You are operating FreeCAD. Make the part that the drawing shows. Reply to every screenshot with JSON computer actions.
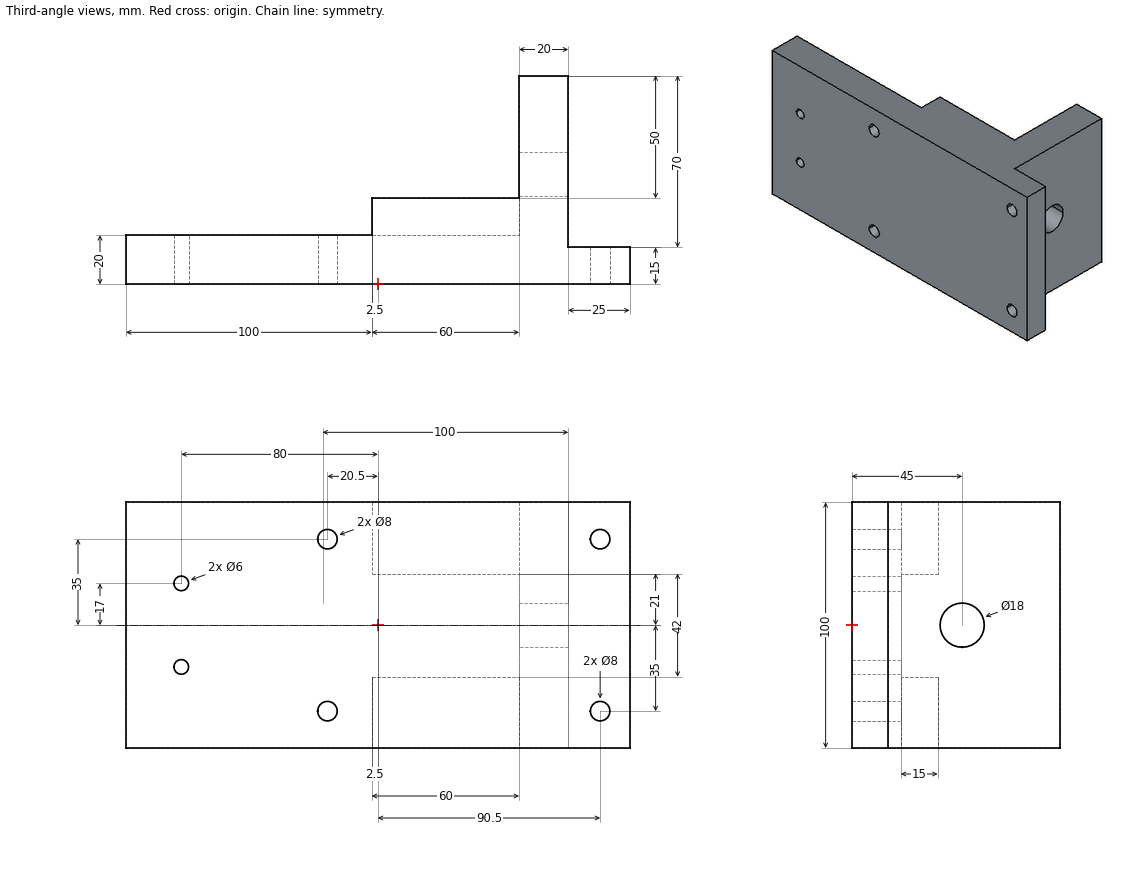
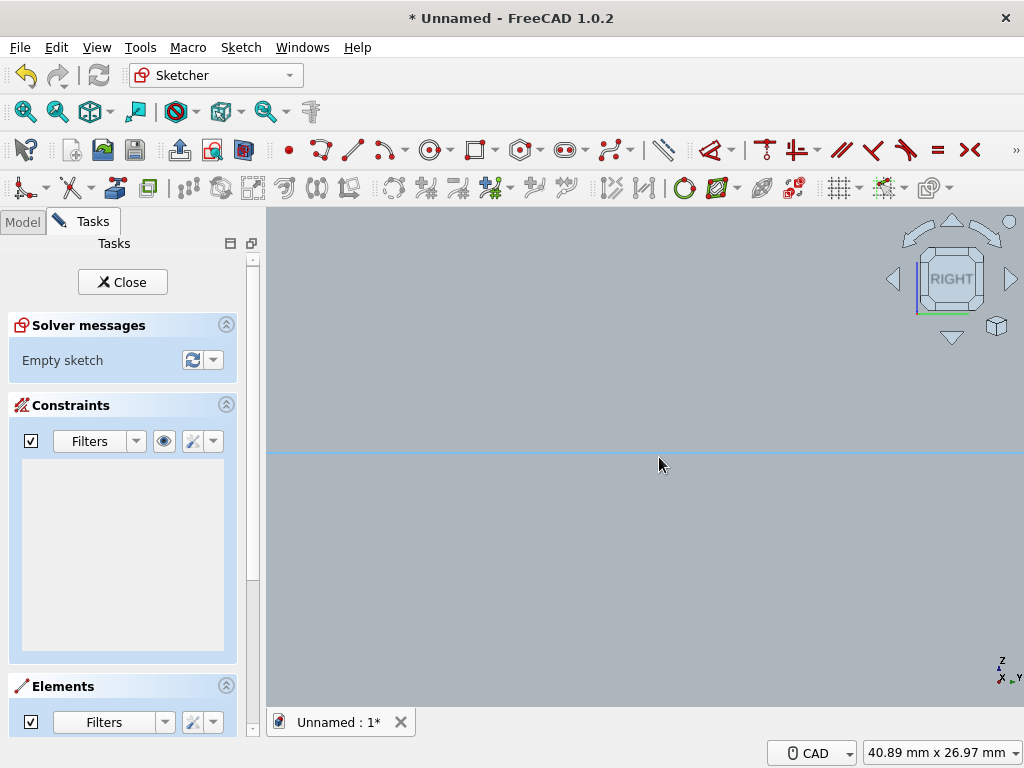
{"action": "left_click", "coordinate": [430, 150]}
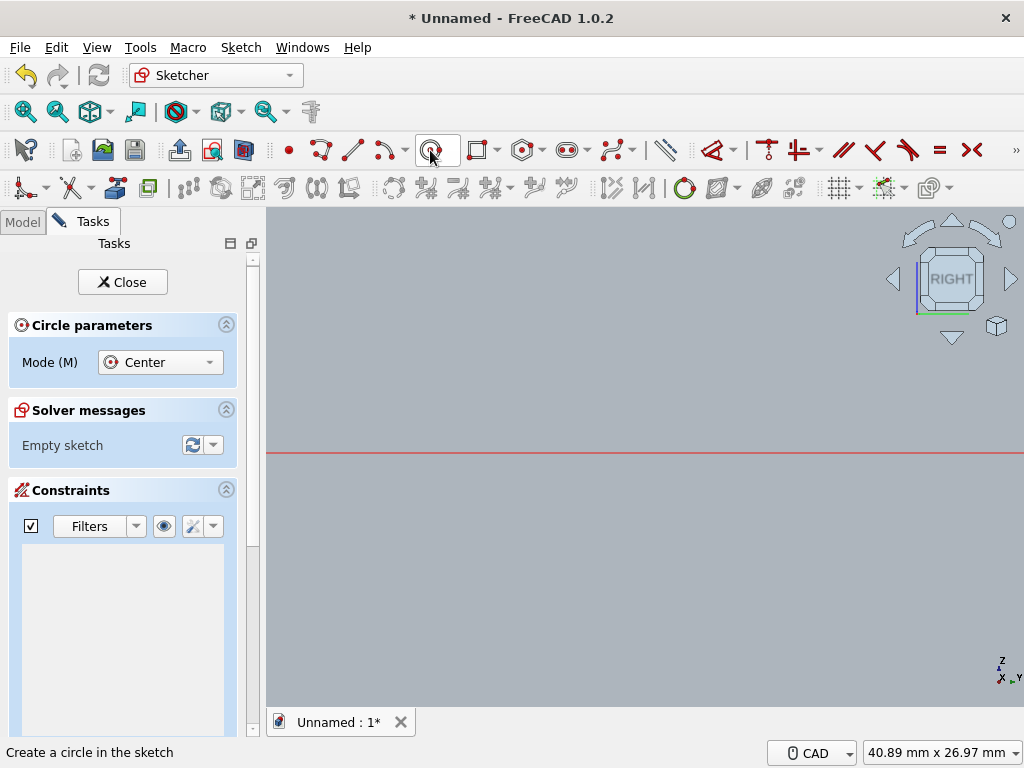
{"action": "left_click", "coordinate": [575, 453]}
{"action": "left_click", "coordinate": [693, 335]}
{"action": "key", "text": "Escape"}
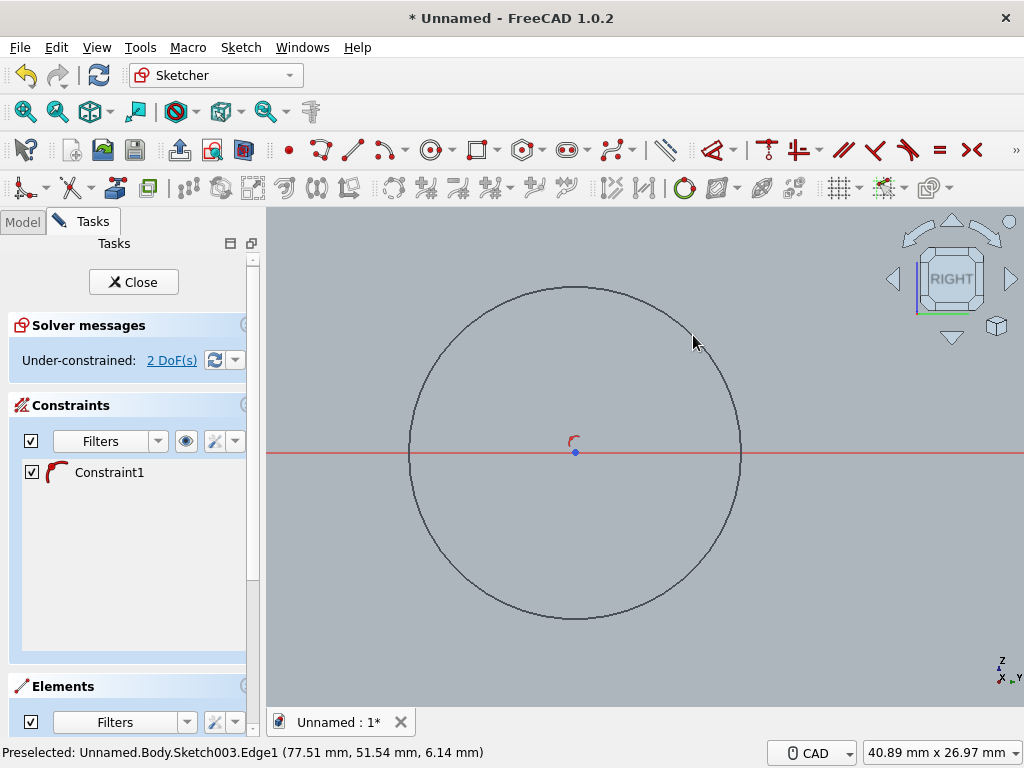
{"action": "left_click", "coordinate": [712, 150]}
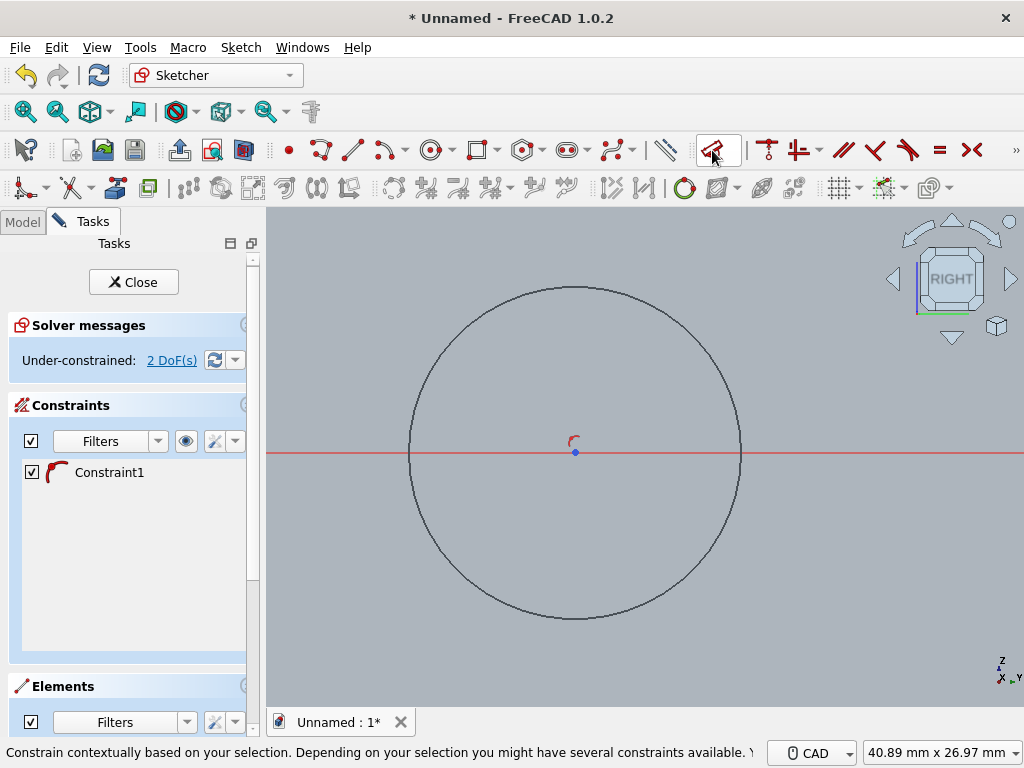
{"action": "left_click", "coordinate": [692, 335]}
{"action": "left_click", "coordinate": [715, 312]}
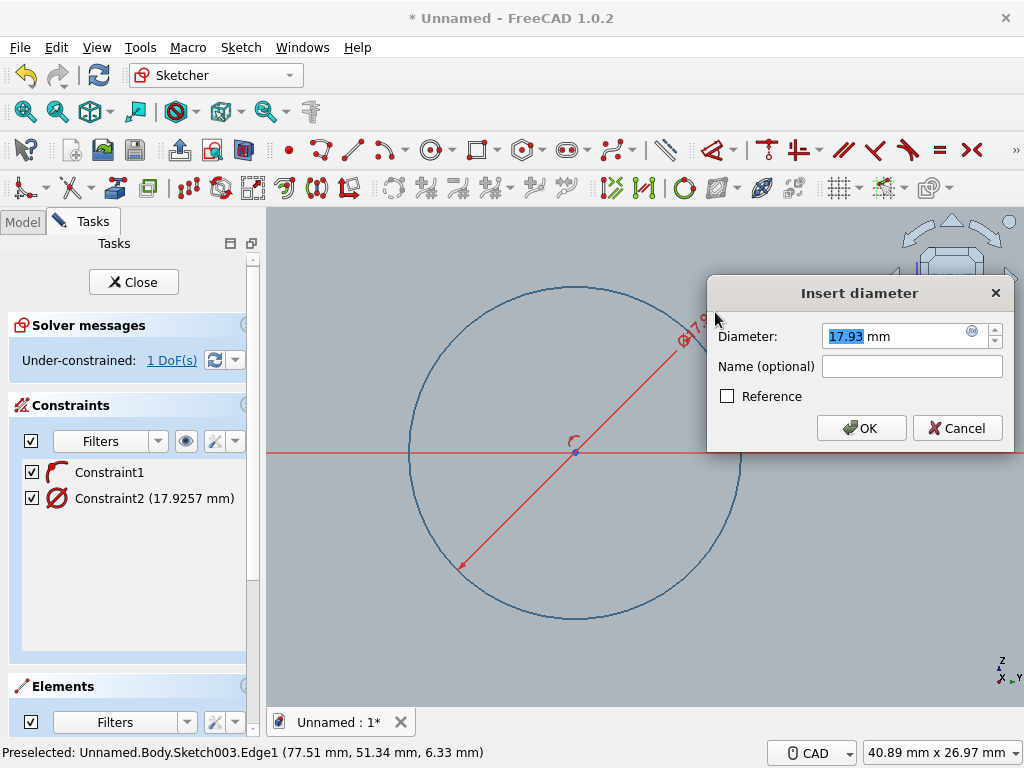
{"action": "type", "text": "18"}
{"action": "key", "text": "Return"}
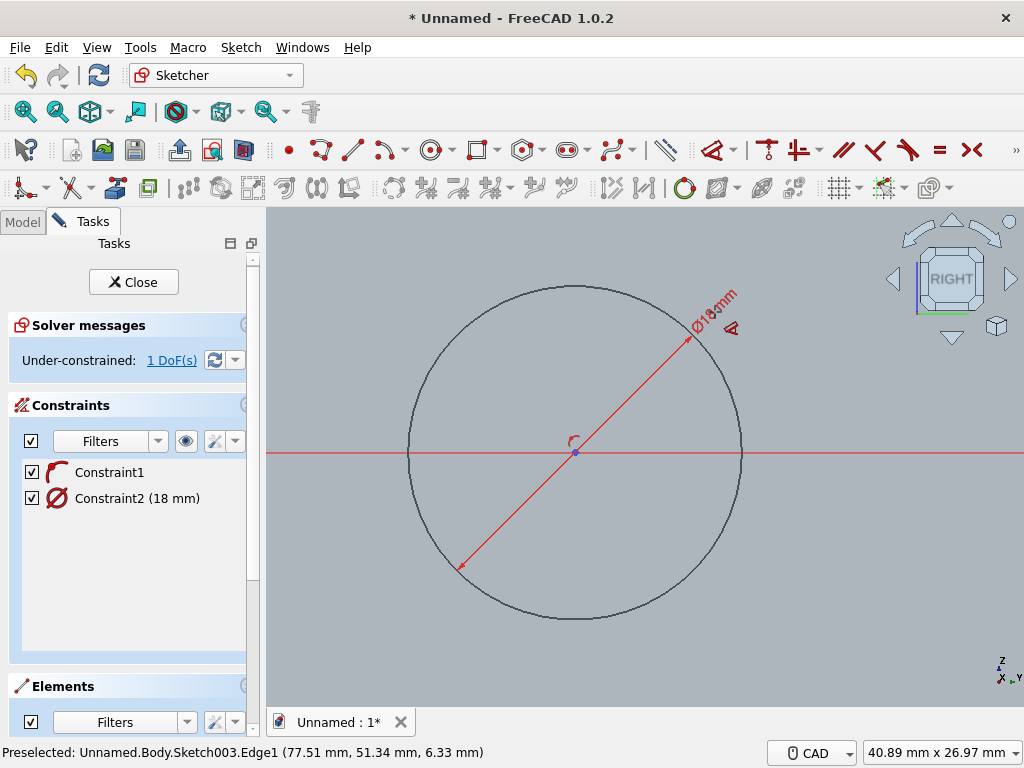
{"action": "left_click", "coordinate": [575, 453]}
{"action": "left_click", "coordinate": [434, 487]}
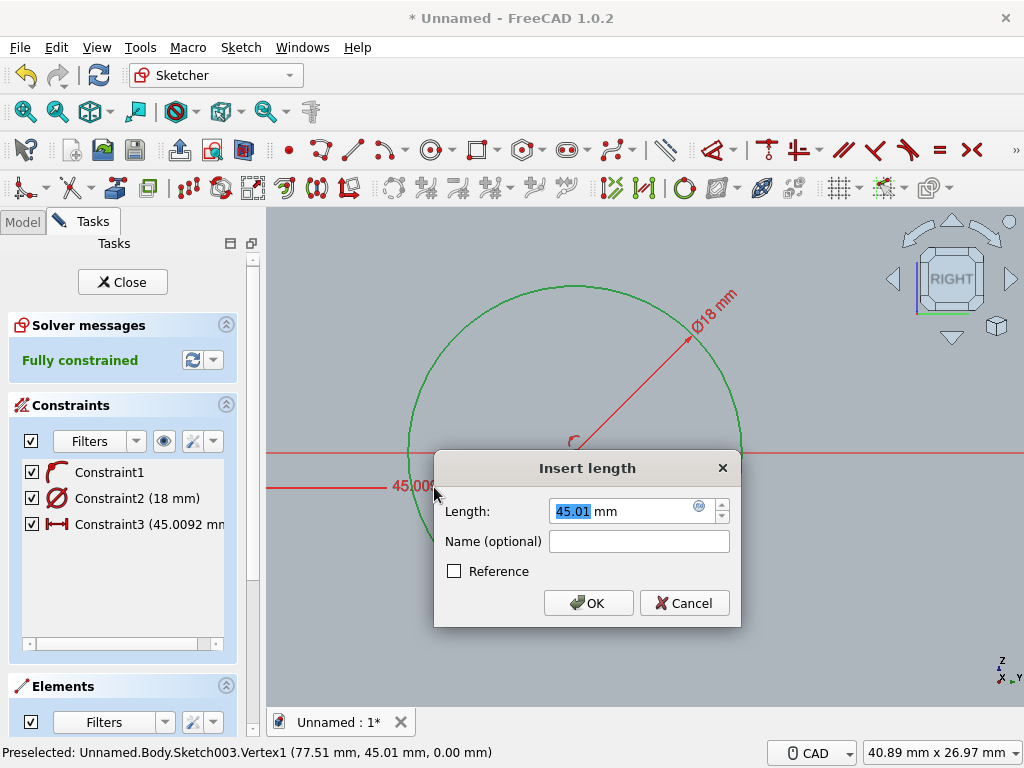
{"action": "type", "text": "45"}
{"action": "key", "text": "Return"}
{"action": "key", "text": "Escape"}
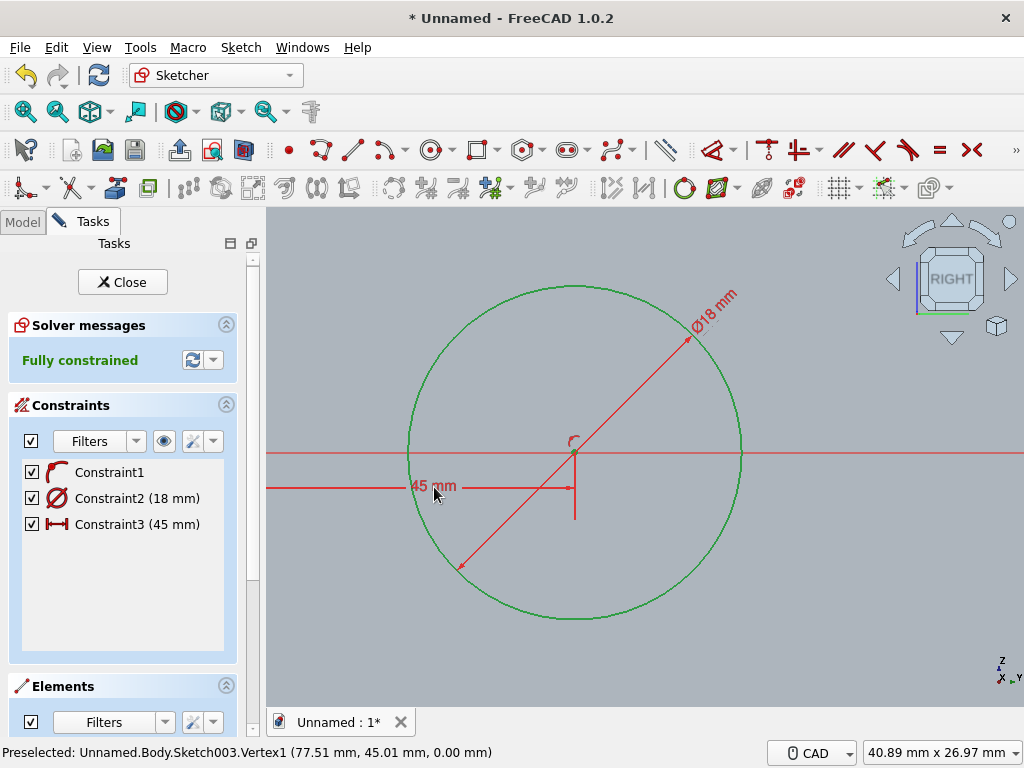
{"action": "left_click", "coordinate": [123, 282]}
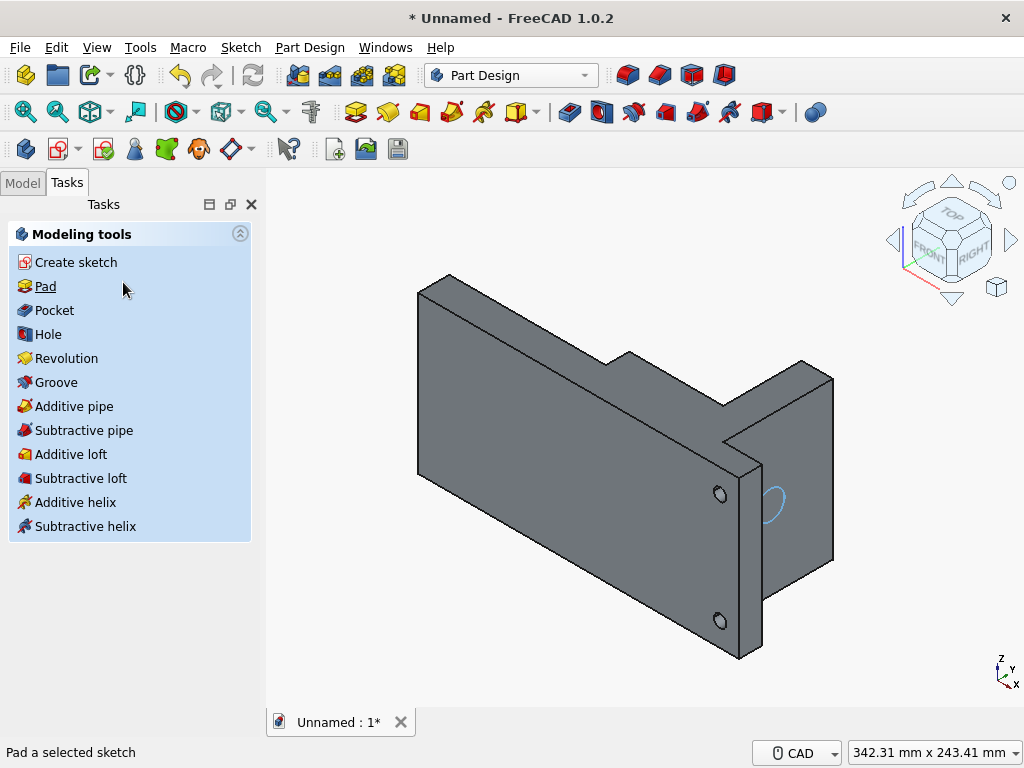
{"action": "left_click", "coordinate": [570, 112]}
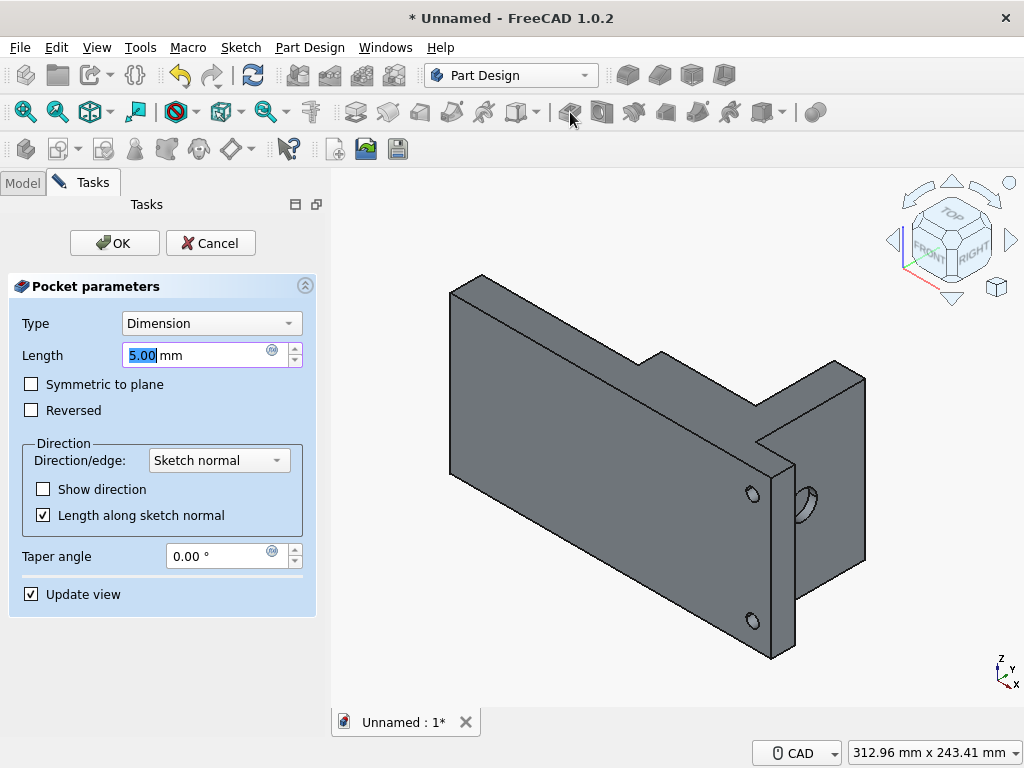
{"action": "type", "text": "100"}
{"action": "key", "text": "Tab"}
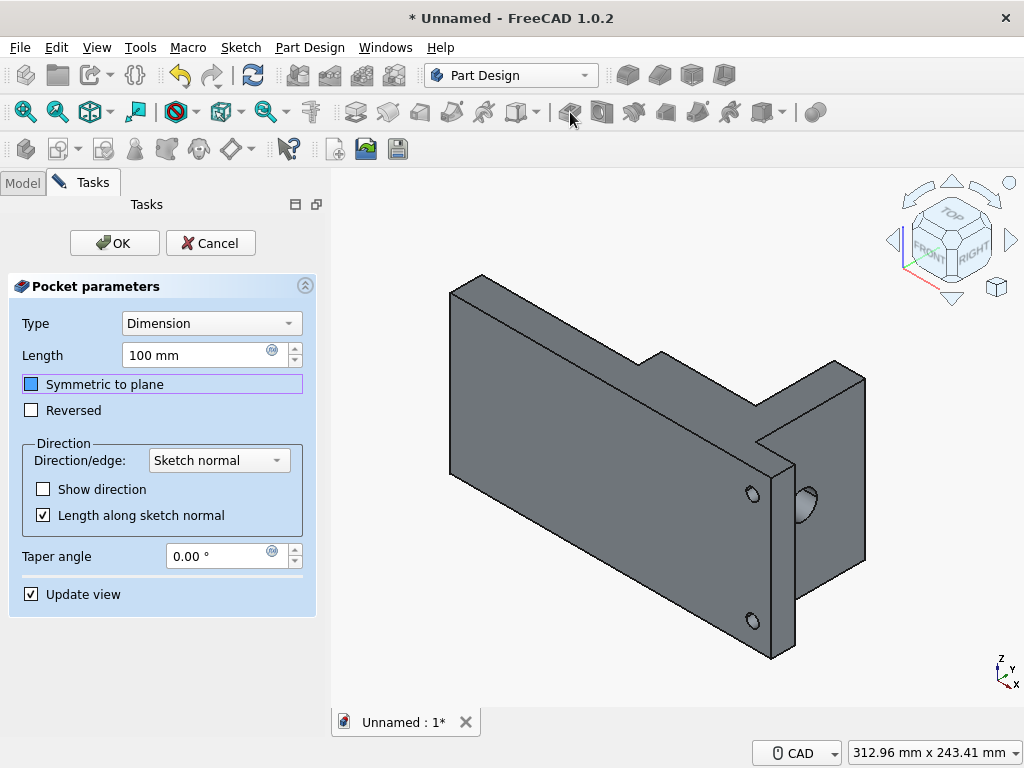
{"action": "left_click", "coordinate": [115, 243]}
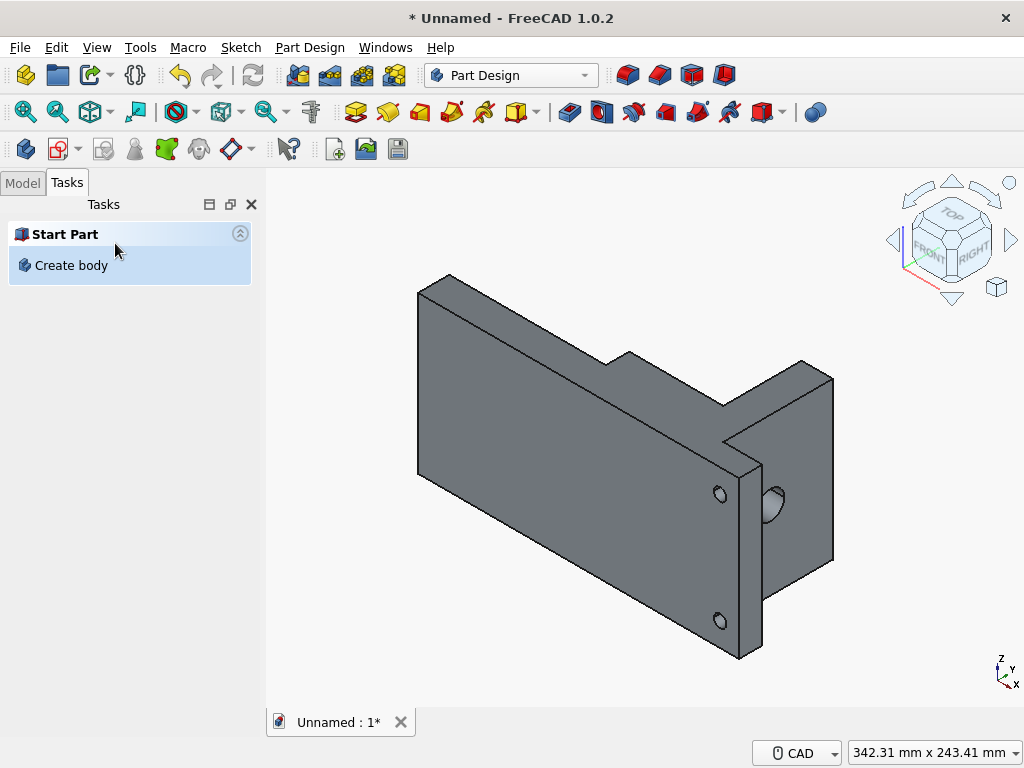
{"action": "key", "text": "4"}